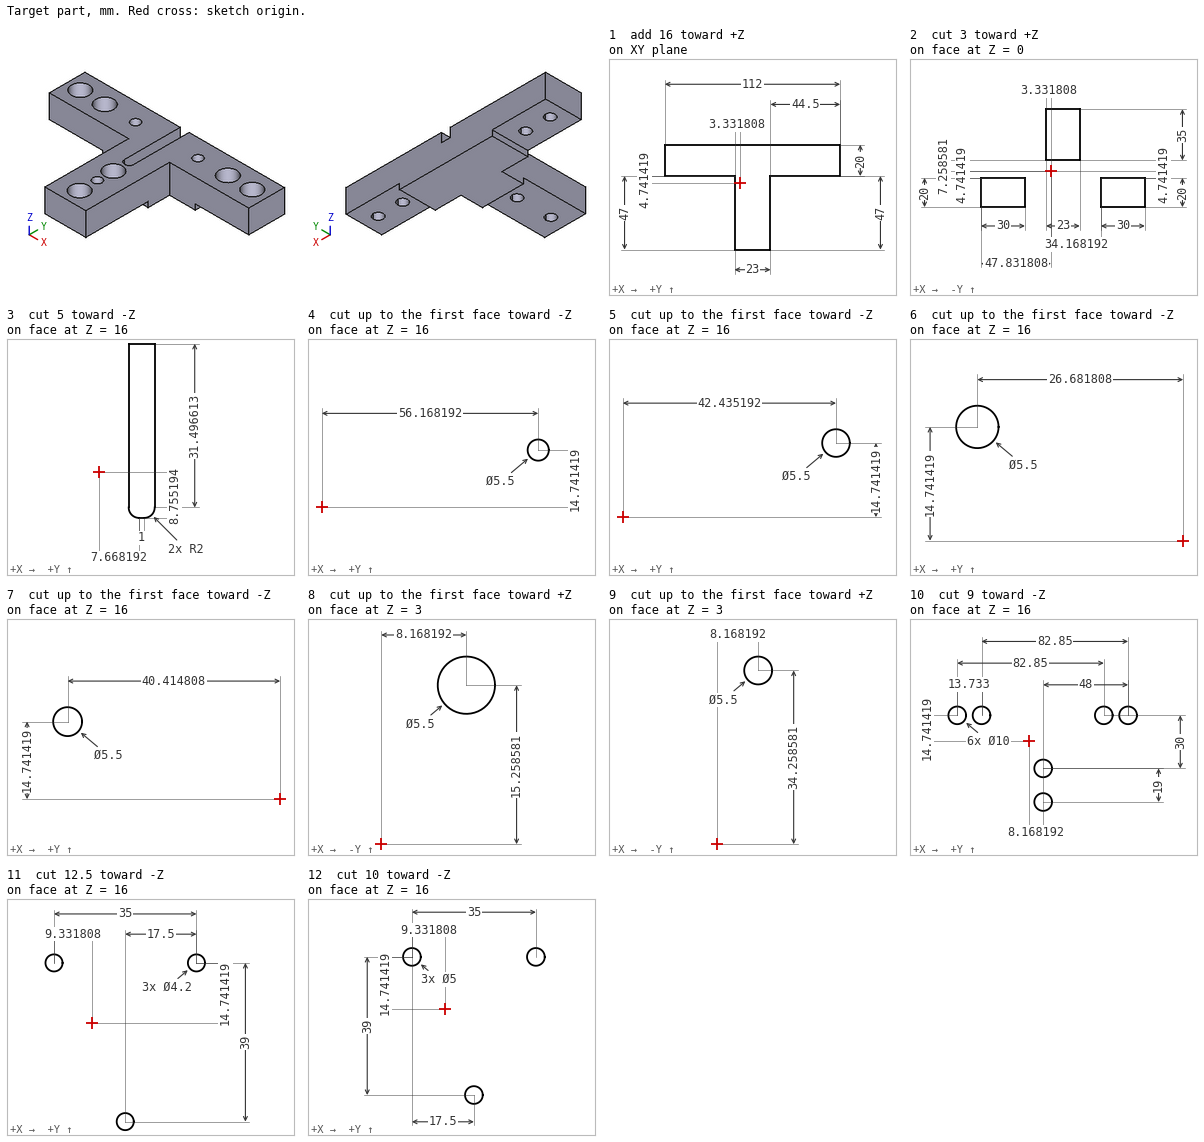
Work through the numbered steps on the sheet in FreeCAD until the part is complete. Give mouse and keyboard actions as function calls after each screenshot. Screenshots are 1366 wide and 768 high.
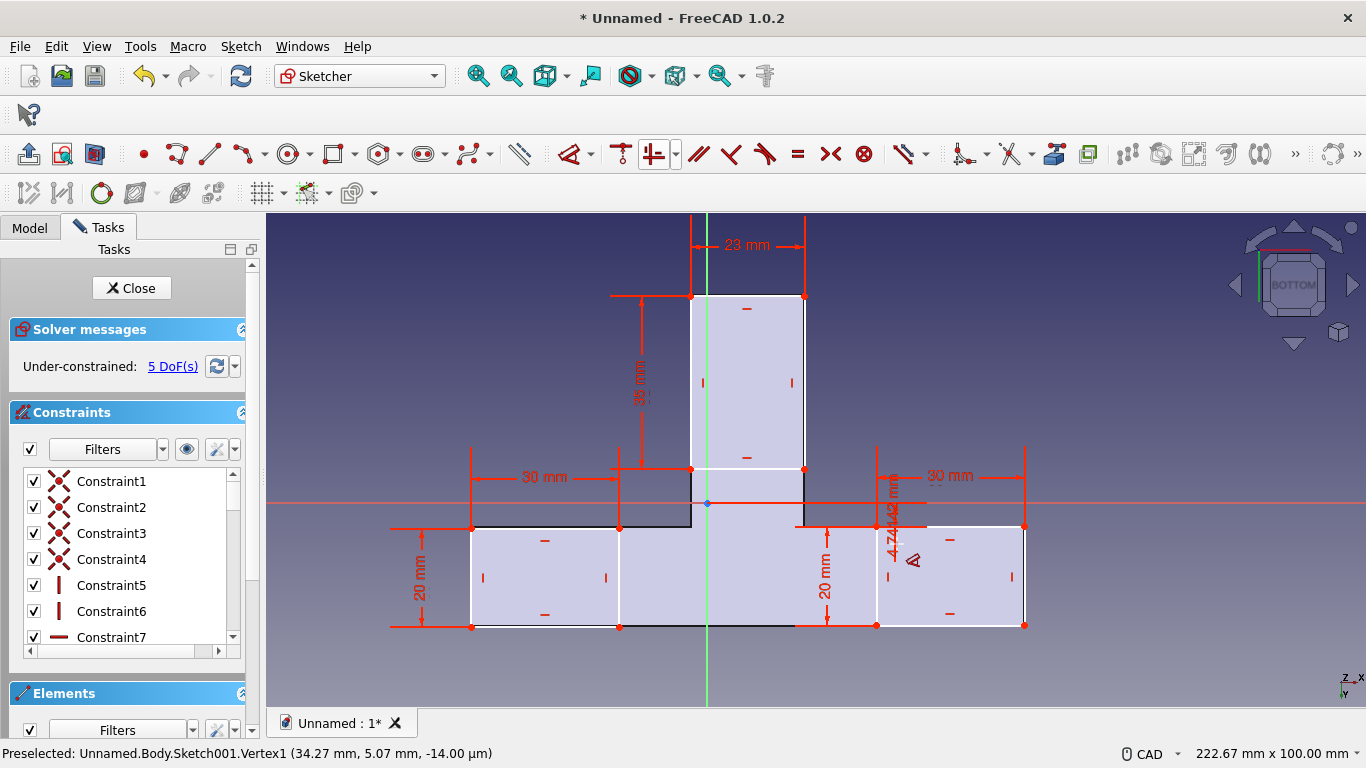
scroll(691, 296, up, 5)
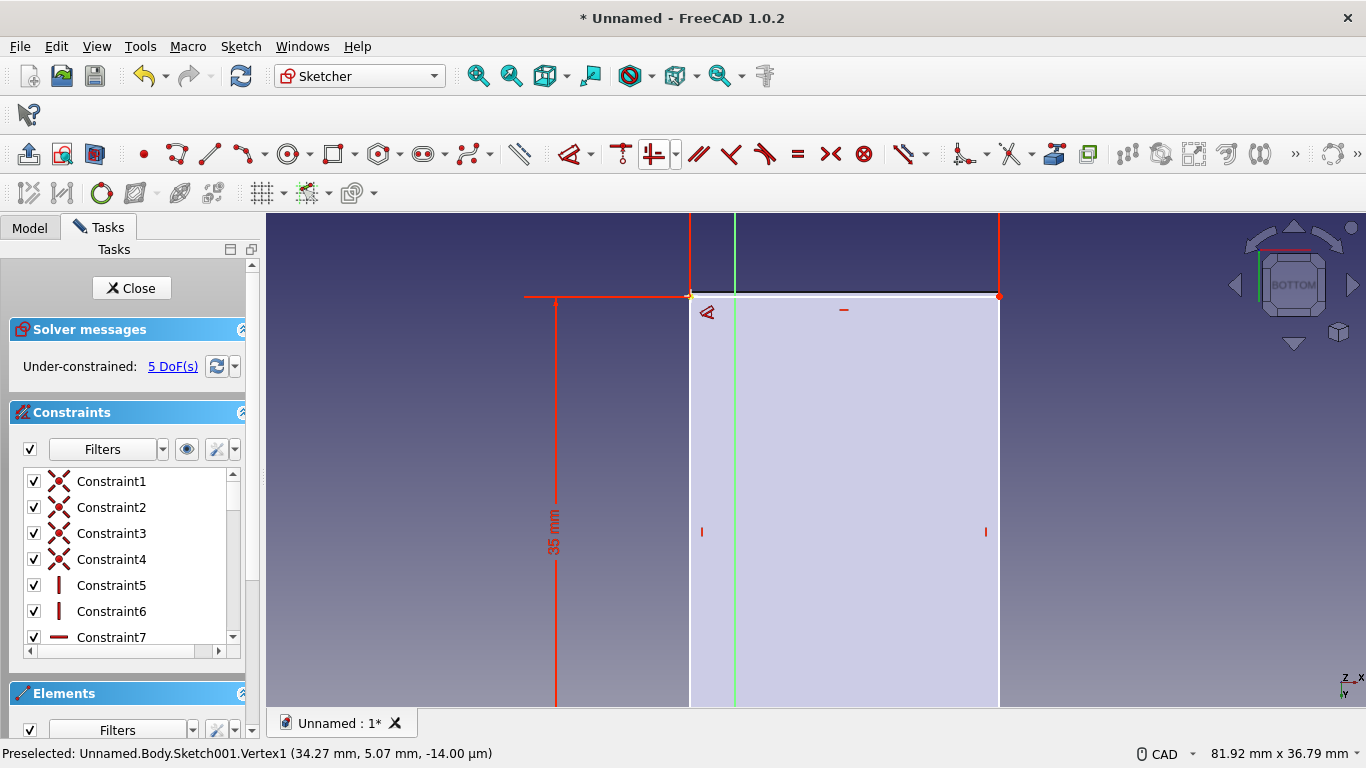
click(690, 297)
click(712, 263)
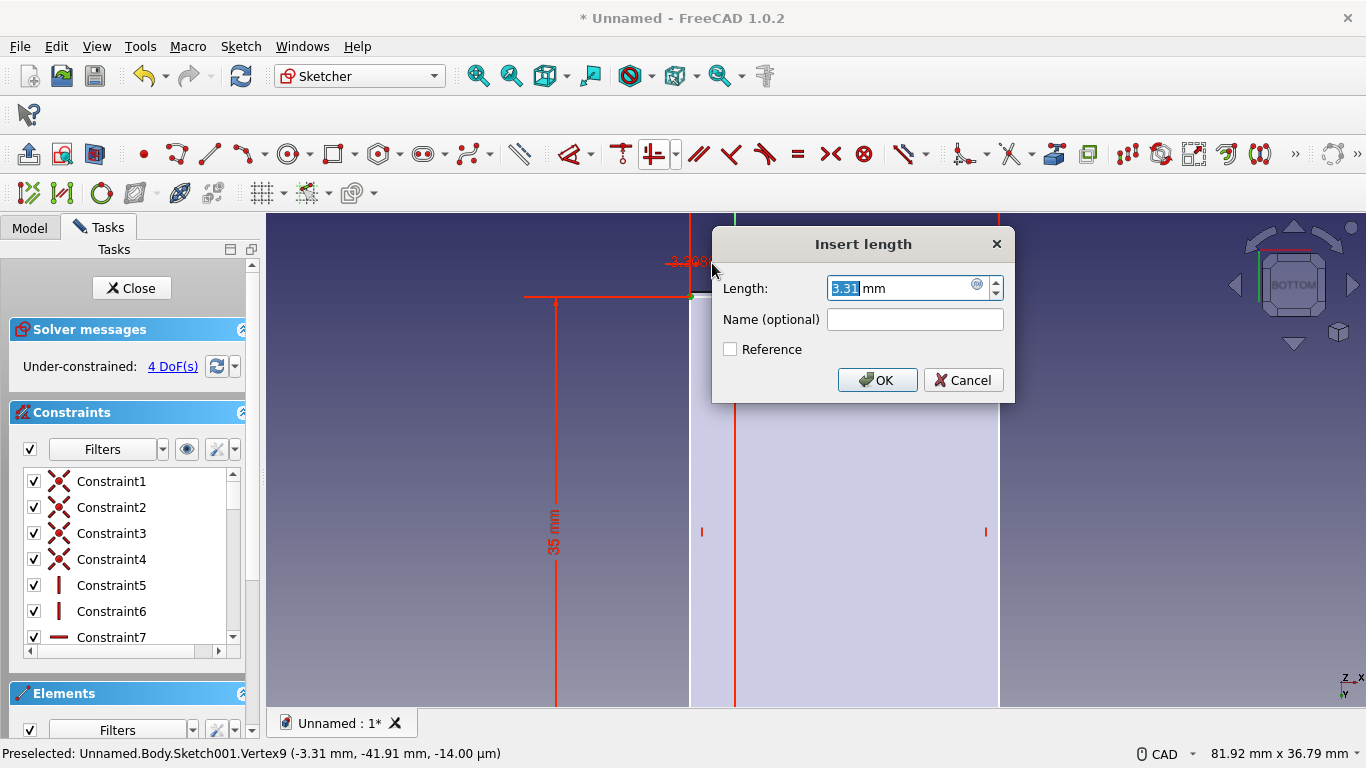
text(3.331808)
key(Return)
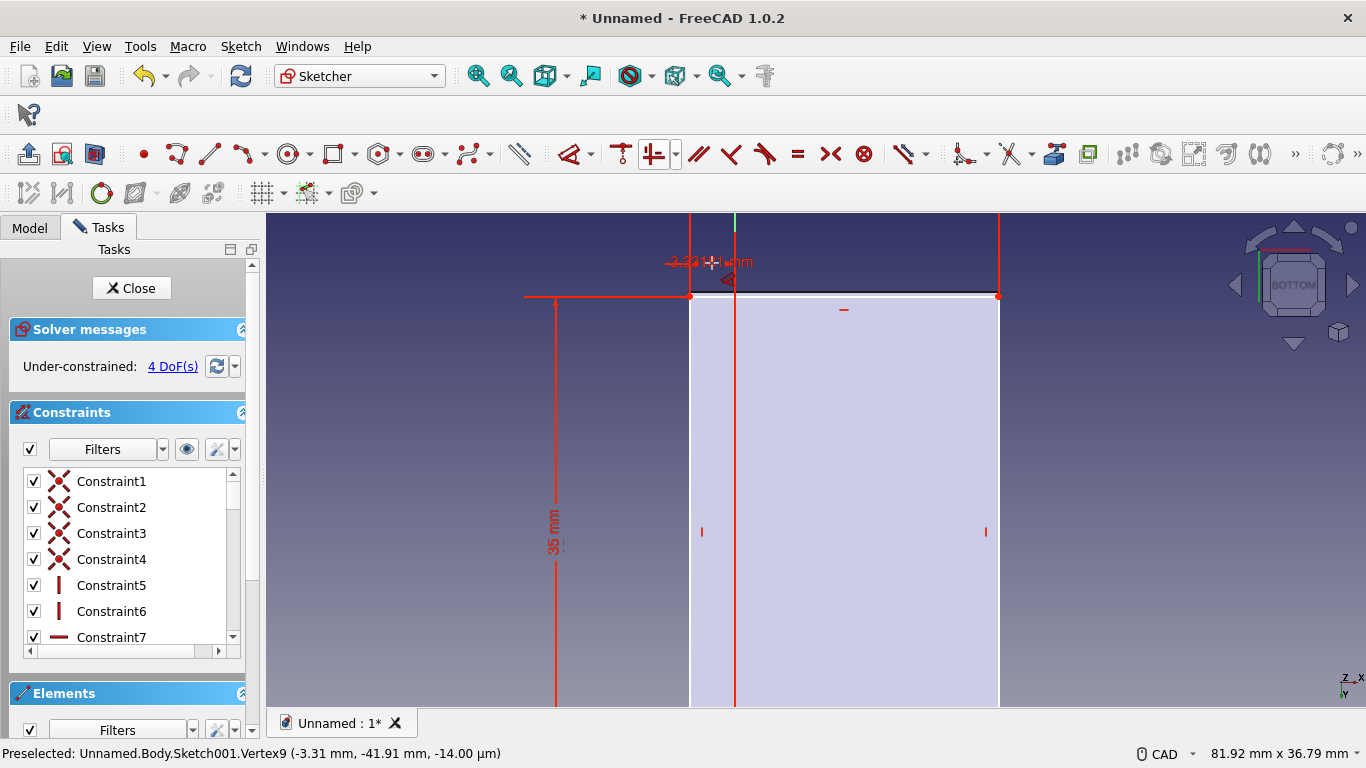
scroll(691, 296, down, 5)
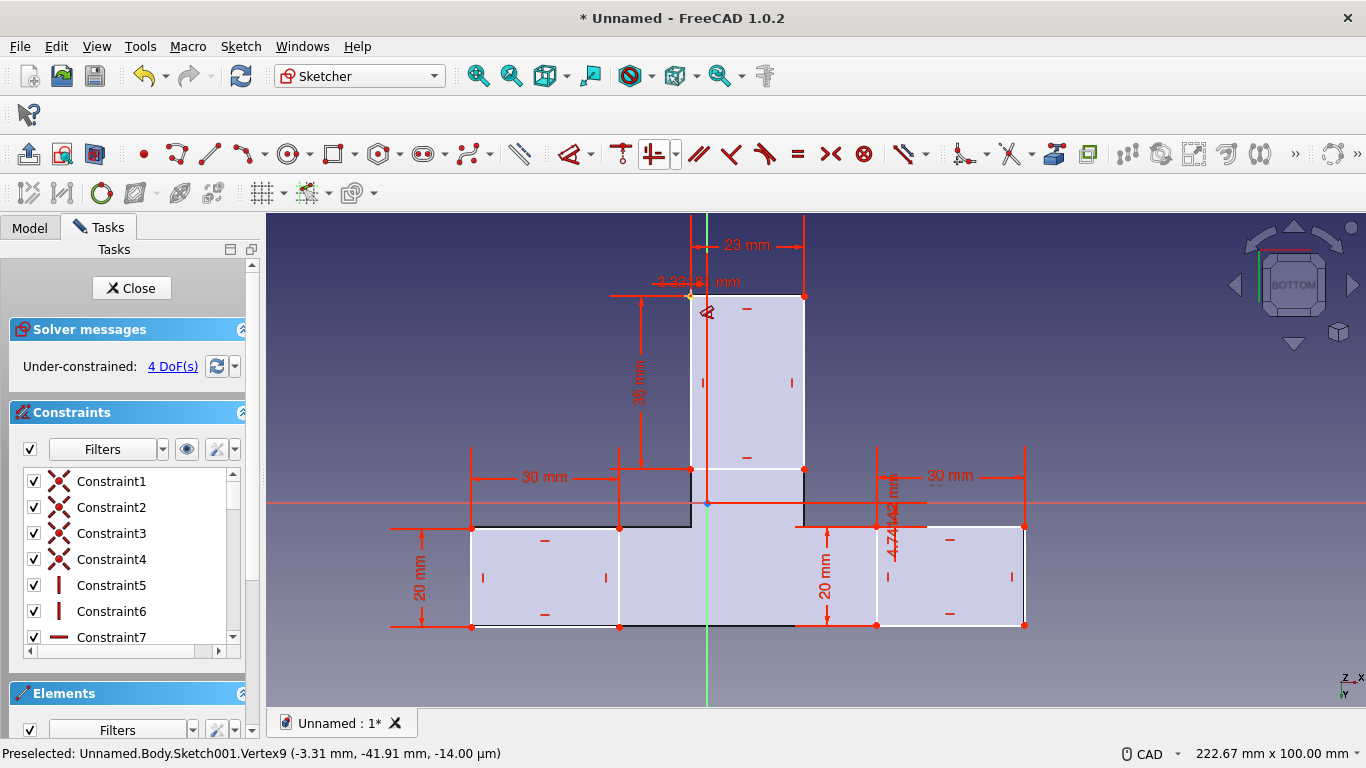
click(691, 469)
click(657, 486)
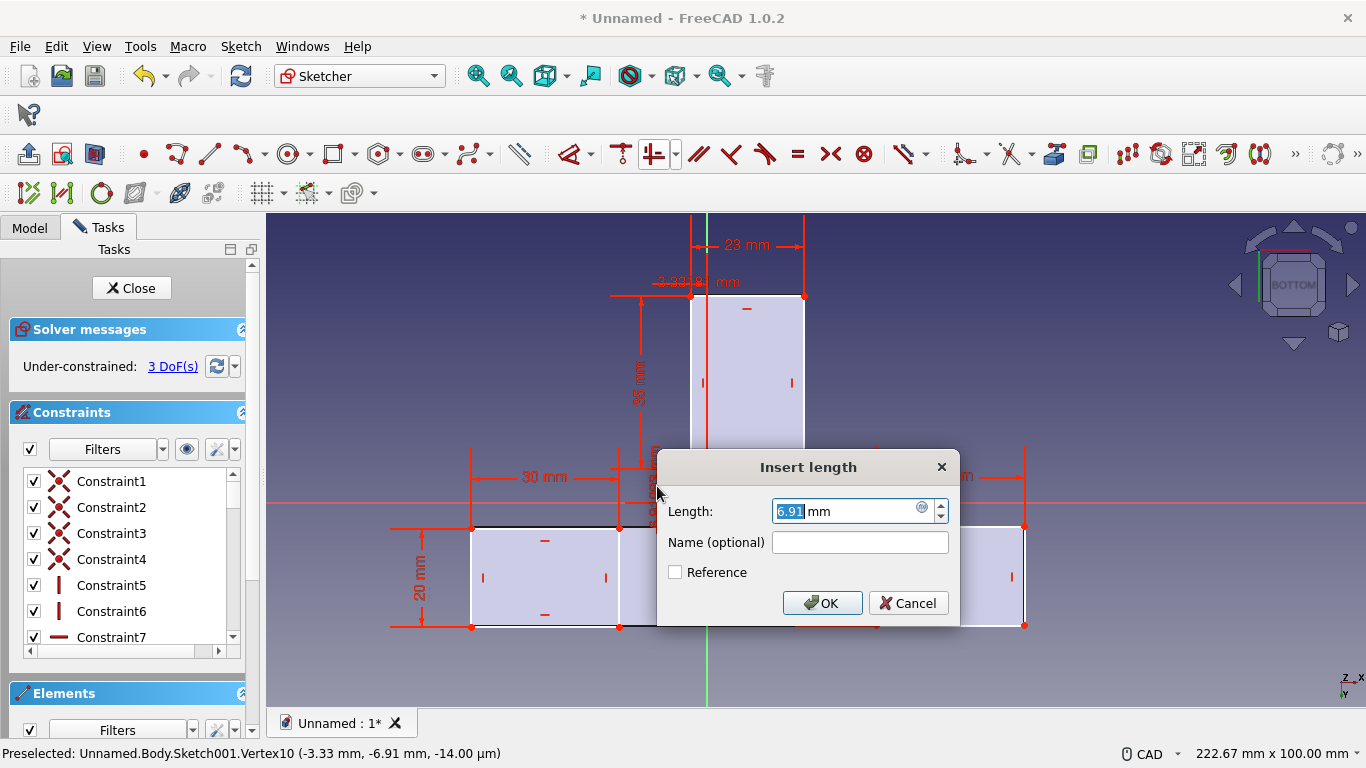
text(7.258581)
key(Return)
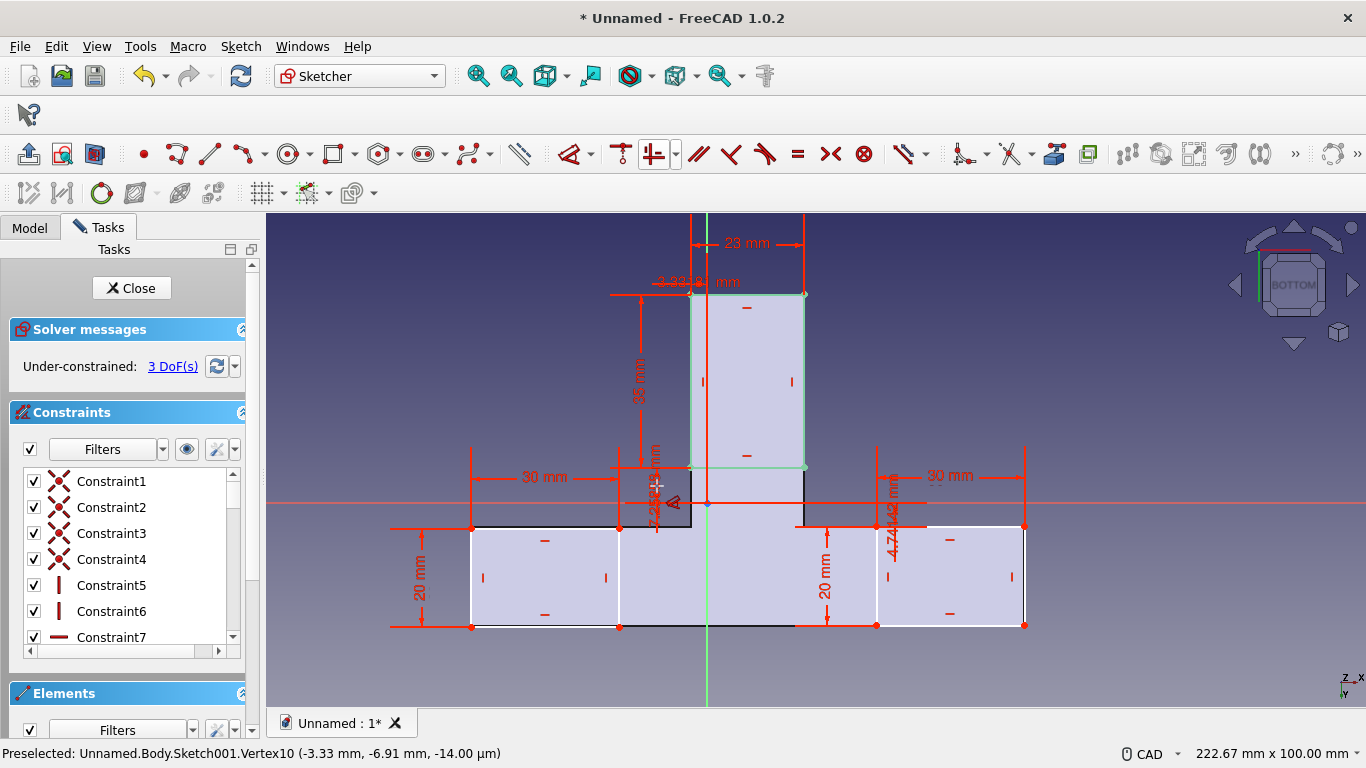
scroll(471, 529, up, 3)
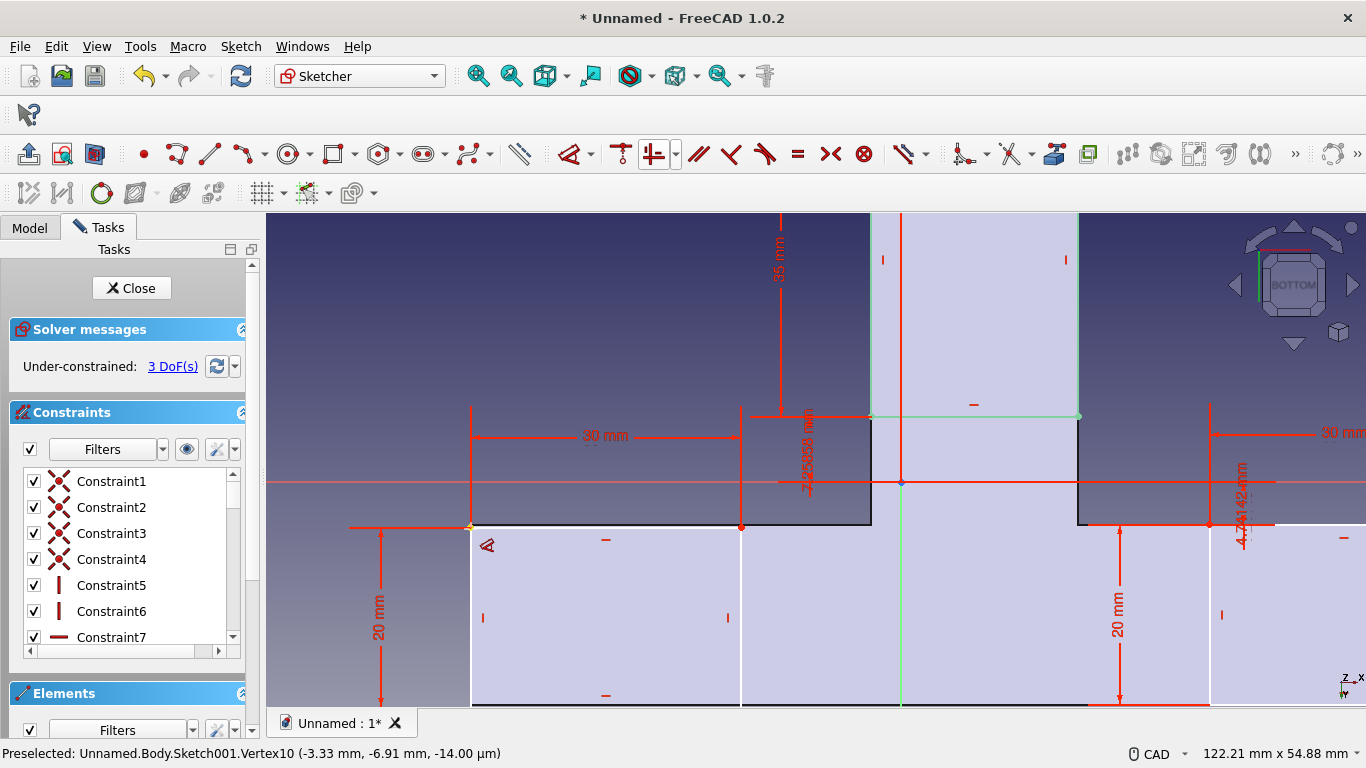
click(471, 528)
click(437, 505)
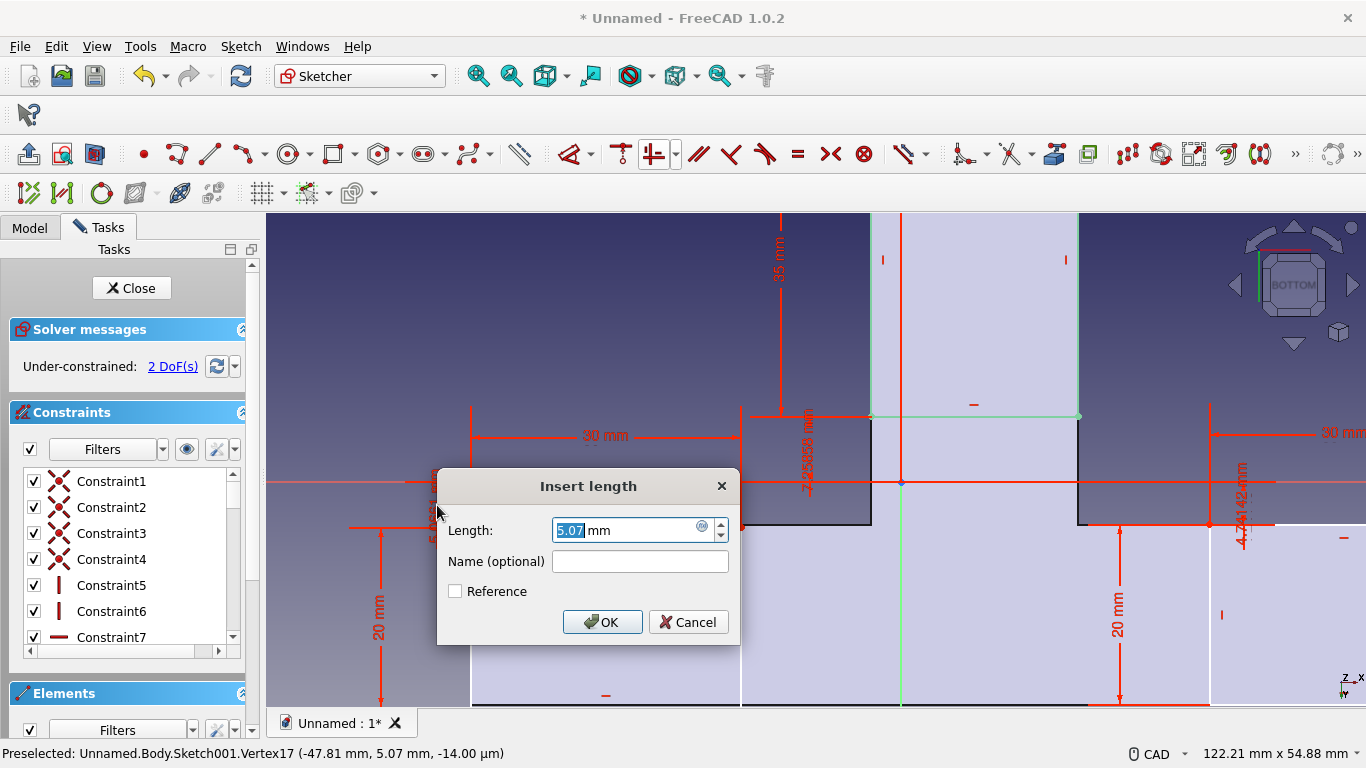
text(4.741419)
key(Return)